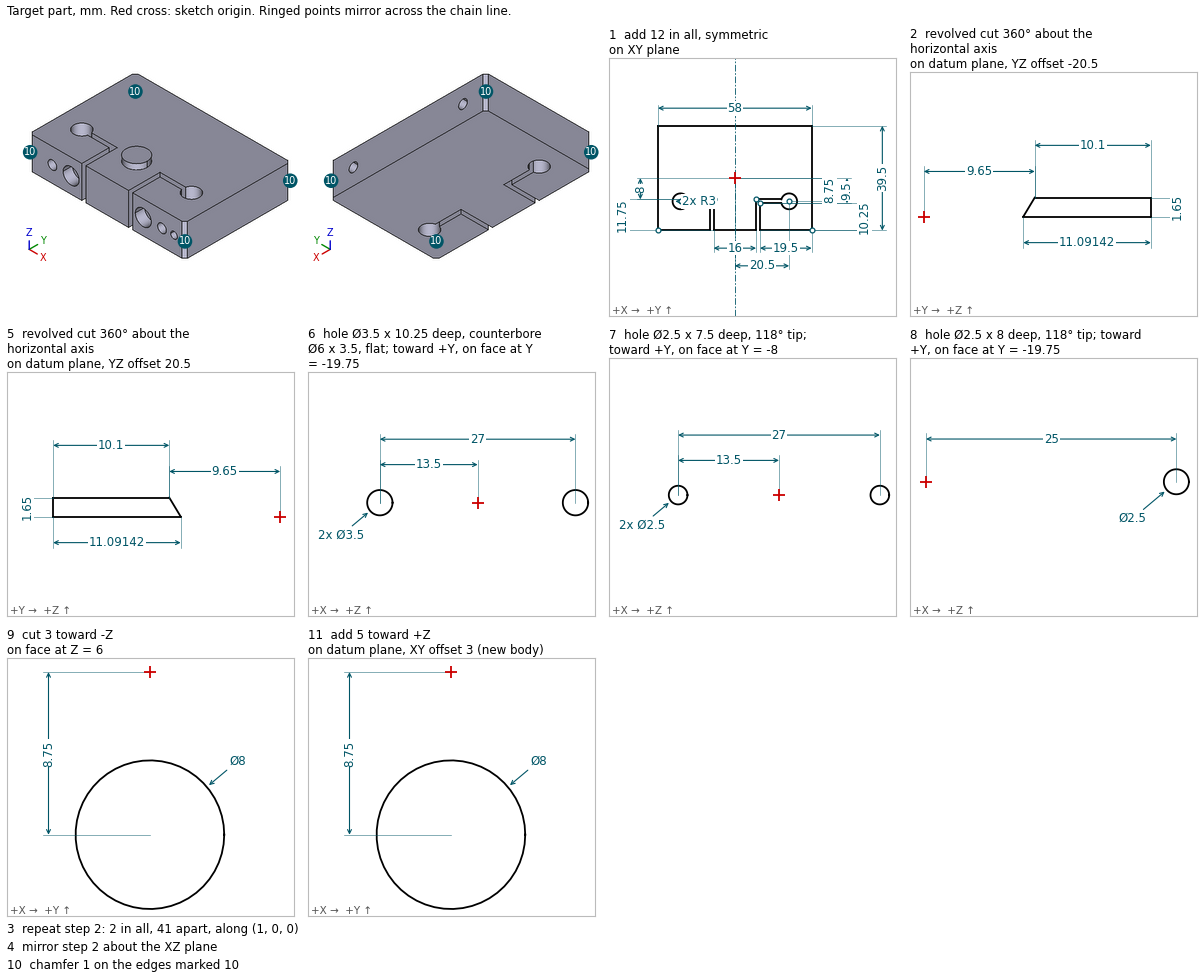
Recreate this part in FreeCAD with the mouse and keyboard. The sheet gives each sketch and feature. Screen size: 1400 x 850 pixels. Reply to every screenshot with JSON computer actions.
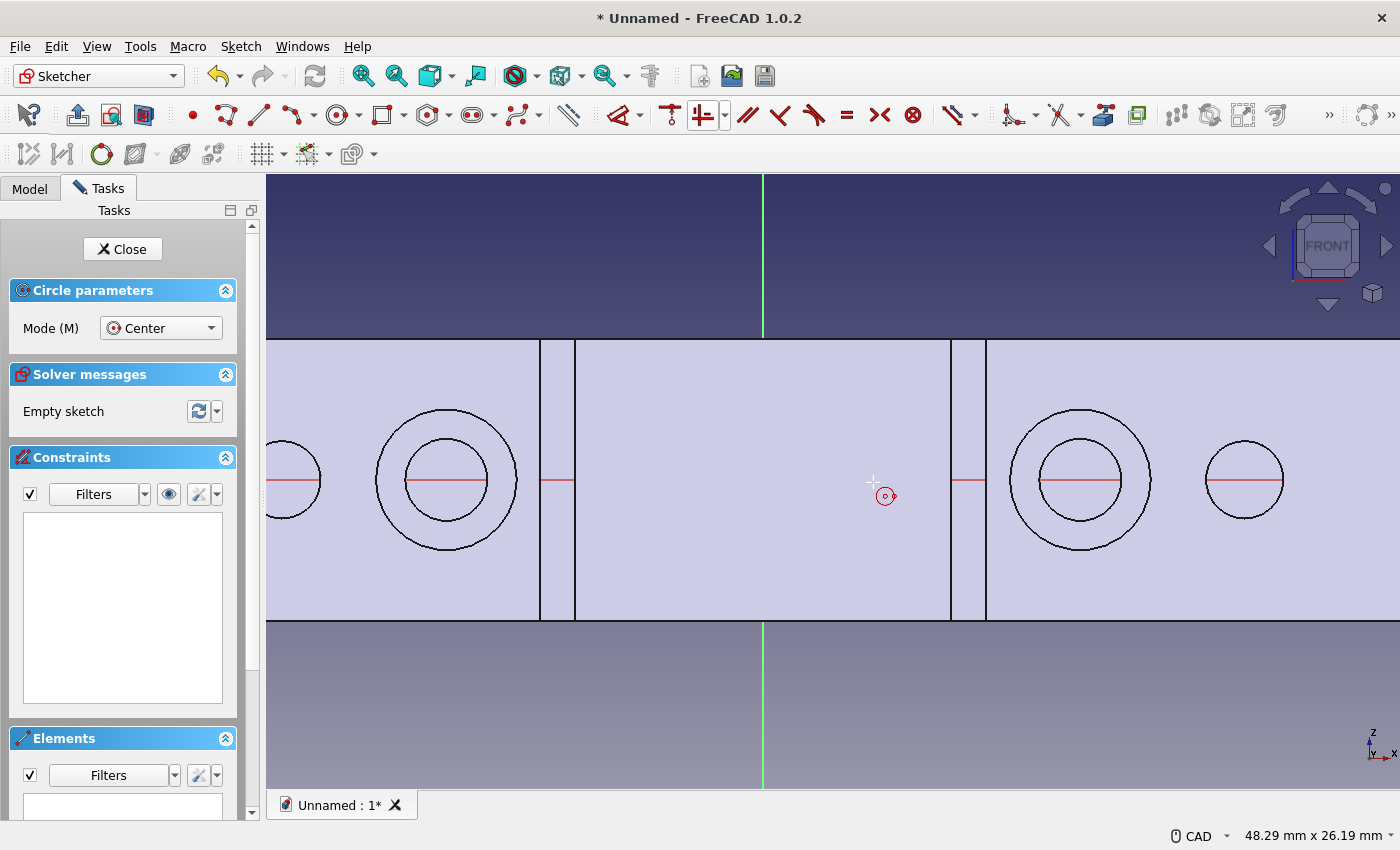
{"action": "left_click", "coordinate": [446, 480]}
{"action": "left_click", "coordinate": [467, 459]}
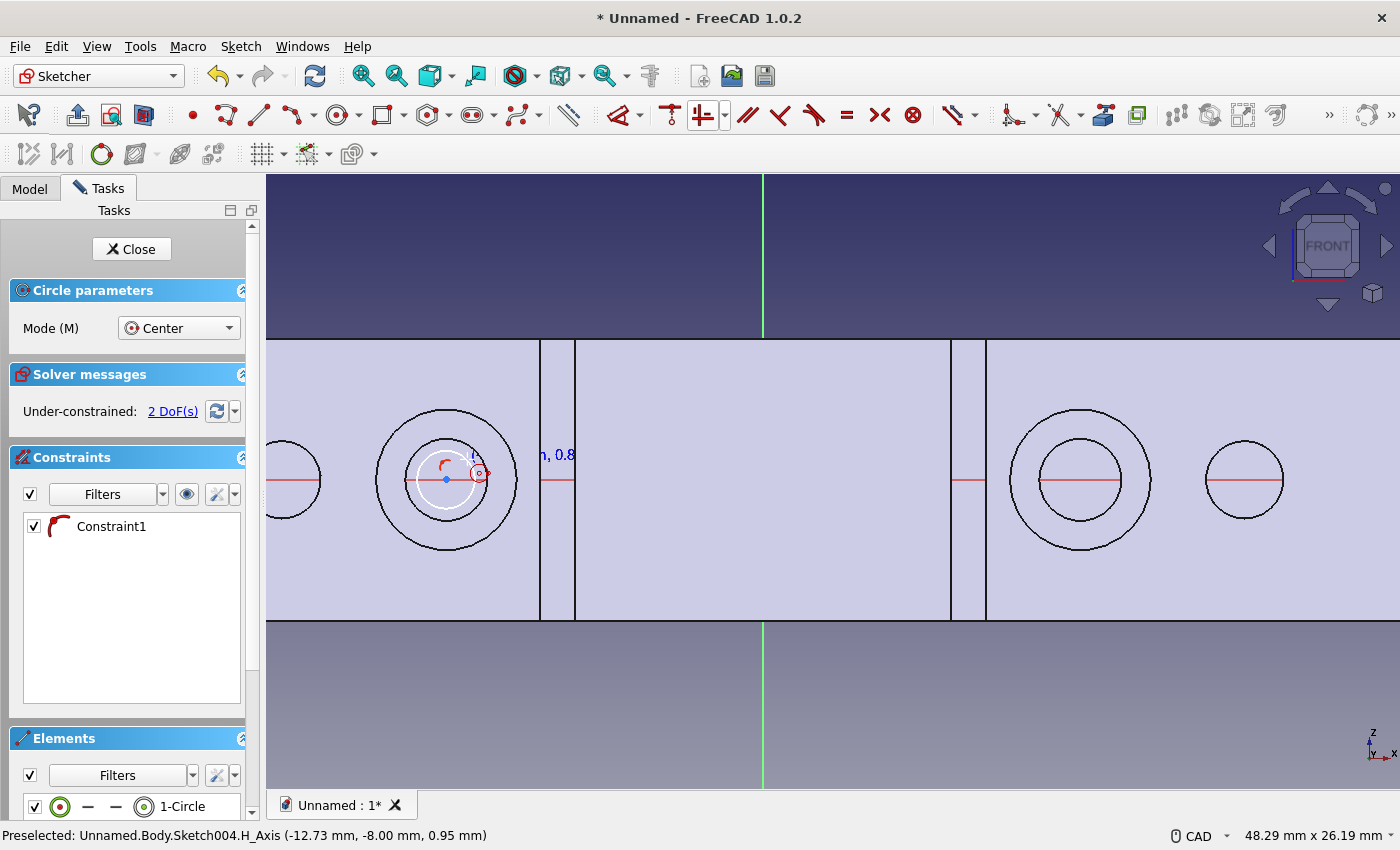
{"action": "left_click", "coordinate": [1080, 480]}
{"action": "left_click", "coordinate": [1101, 459]}
{"action": "key", "text": "Escape"}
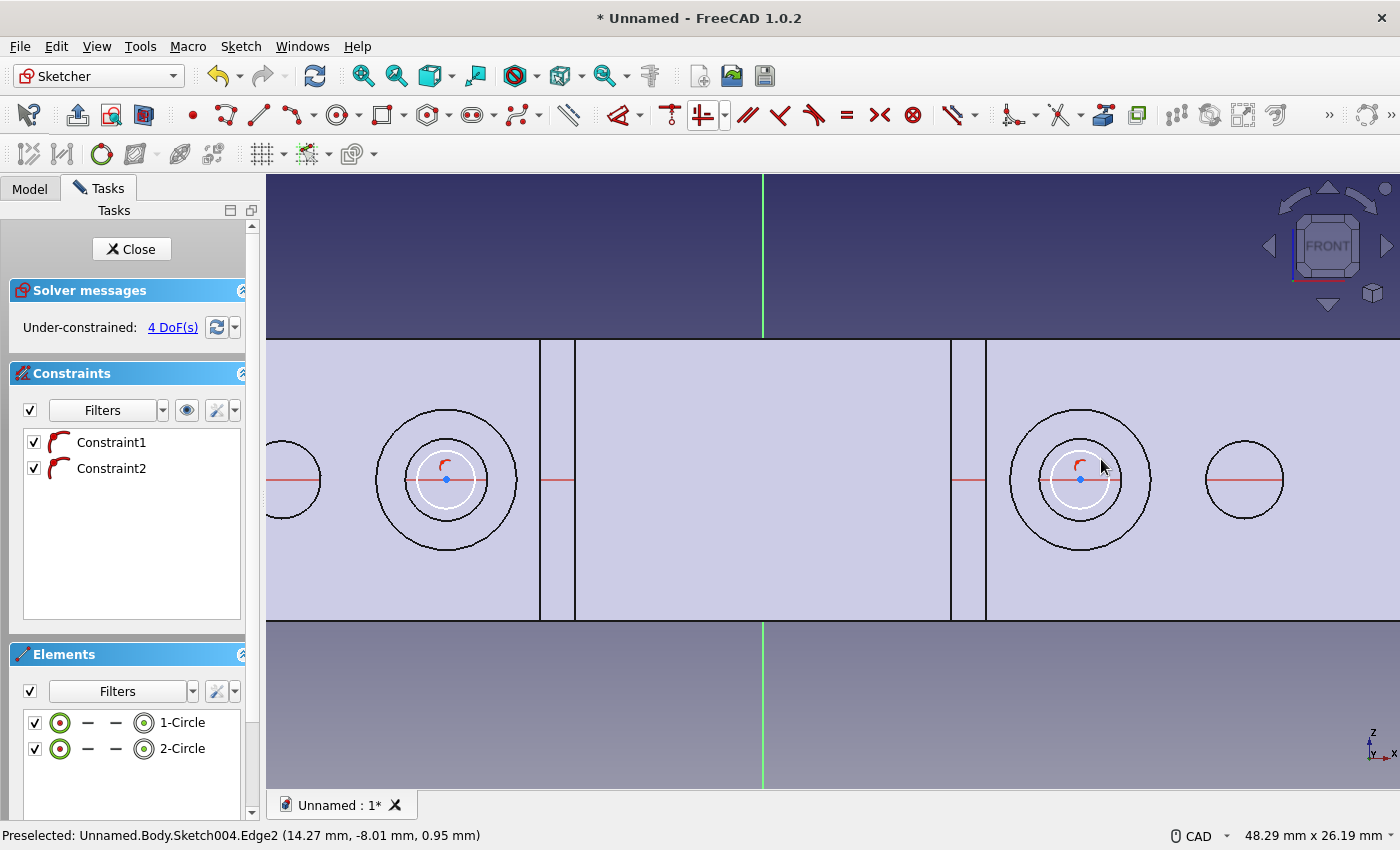
{"action": "left_click", "coordinate": [466, 459]}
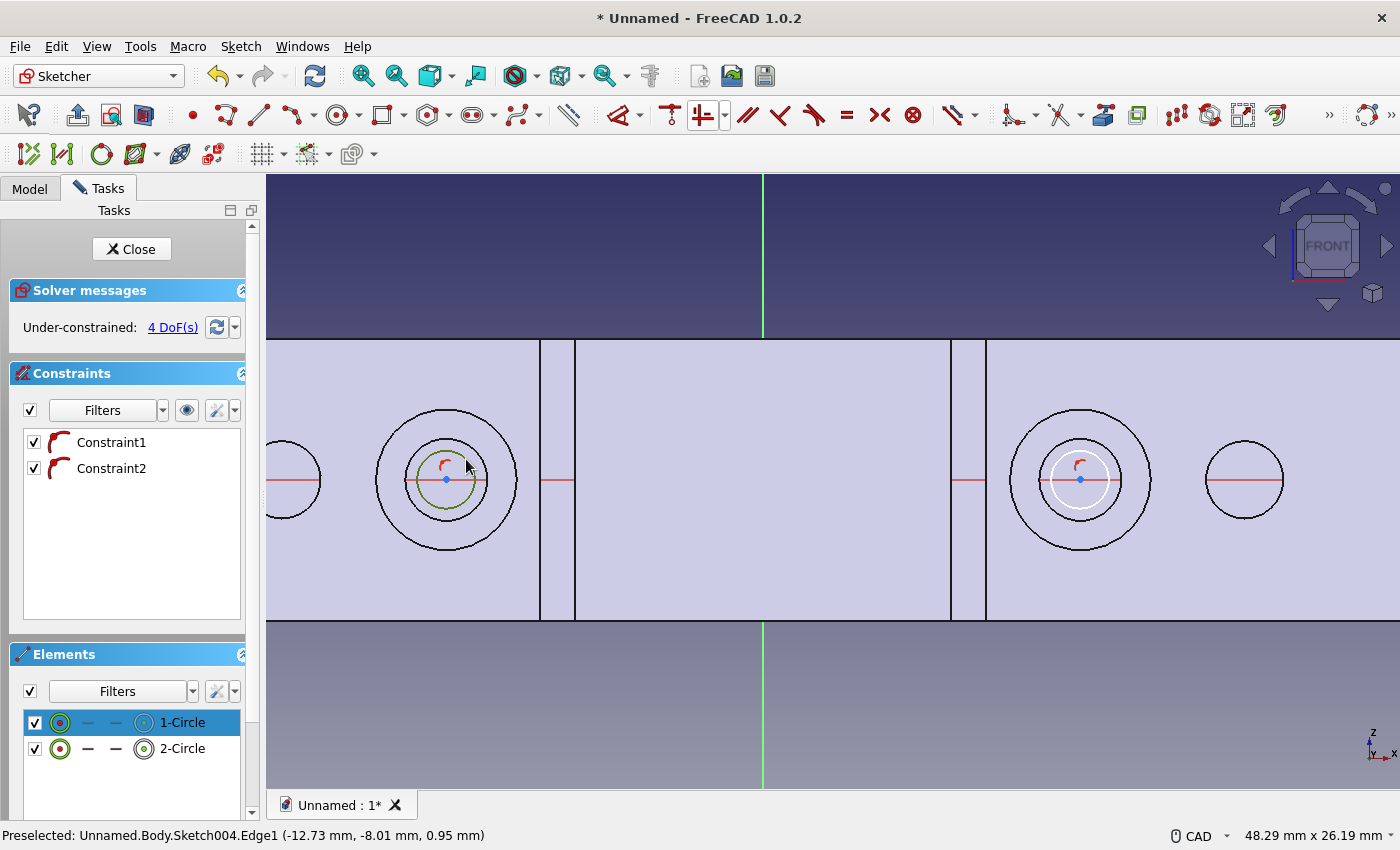
{"action": "left_click", "coordinate": [1100, 459]}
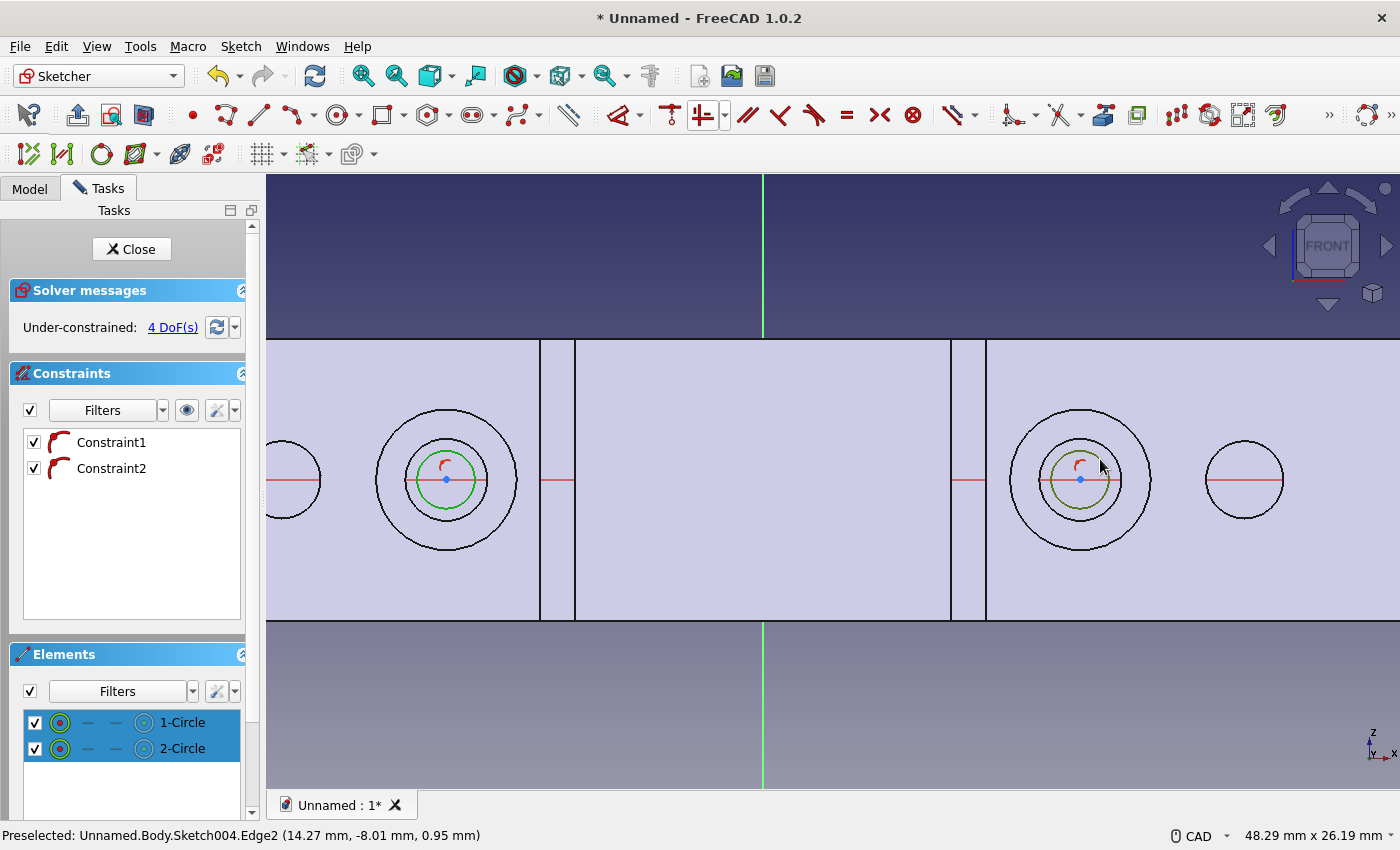
{"action": "left_click", "coordinate": [847, 116]}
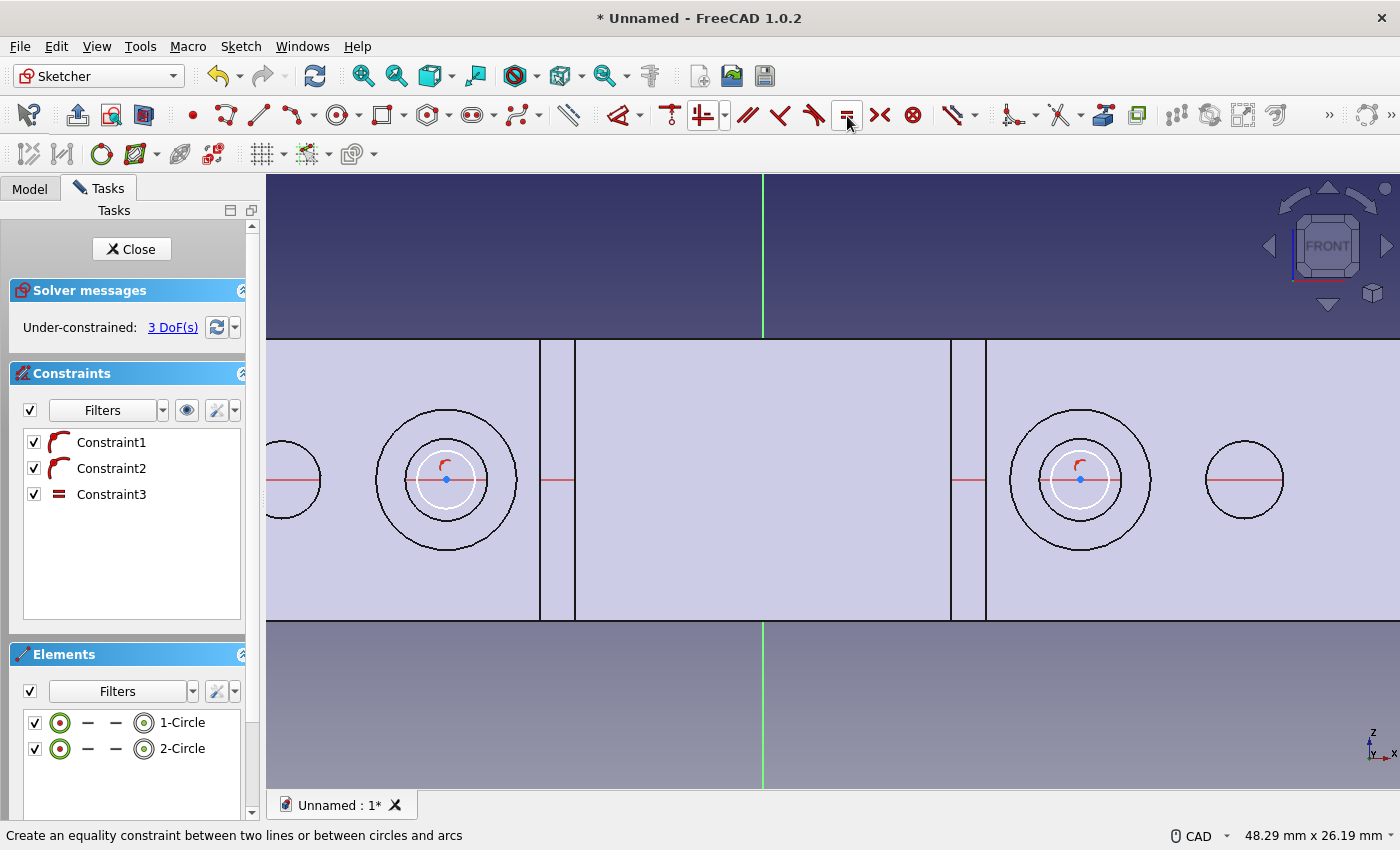
{"action": "left_click", "coordinate": [618, 116]}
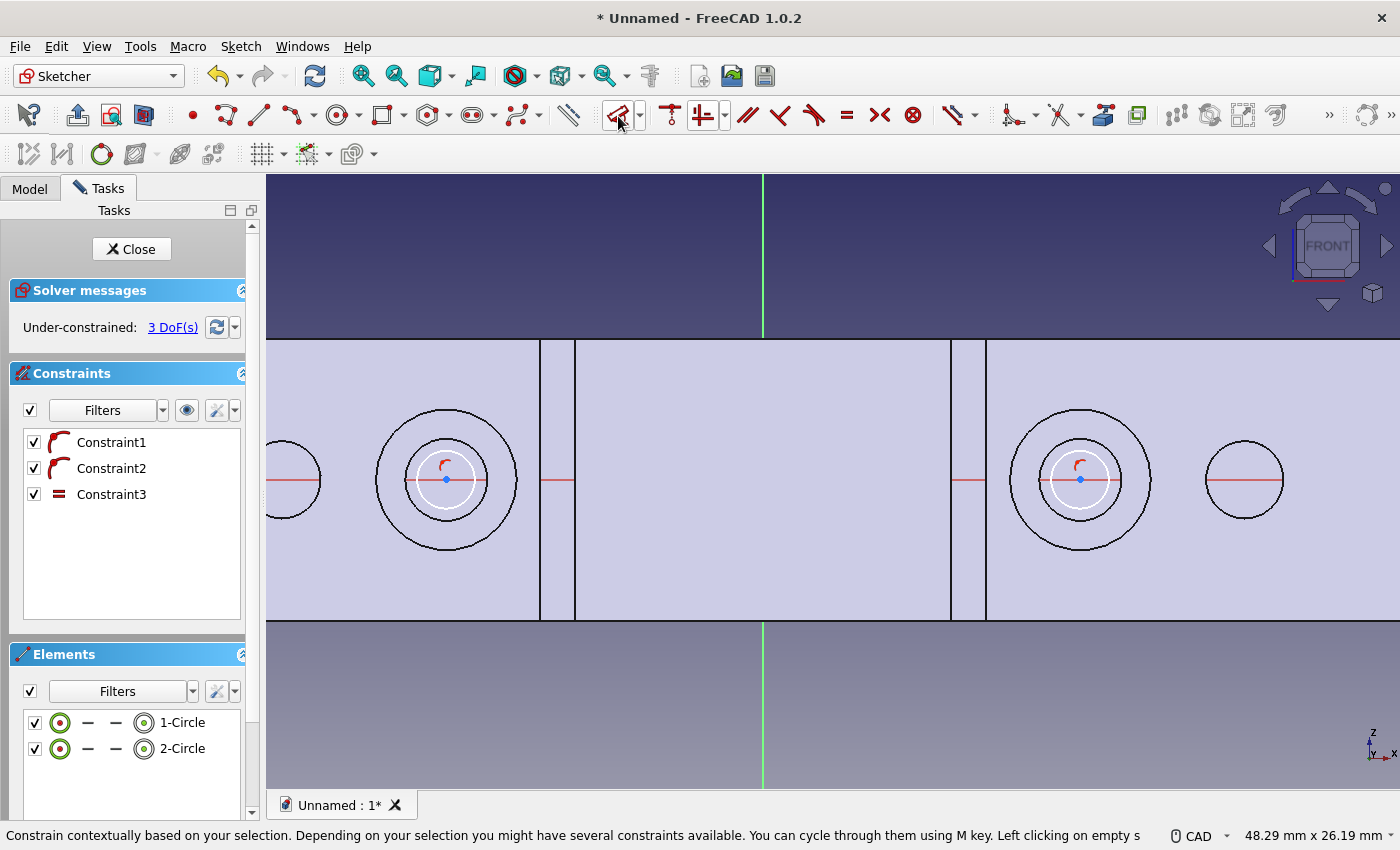
{"action": "left_click", "coordinate": [466, 459]}
{"action": "left_click", "coordinate": [488, 436]}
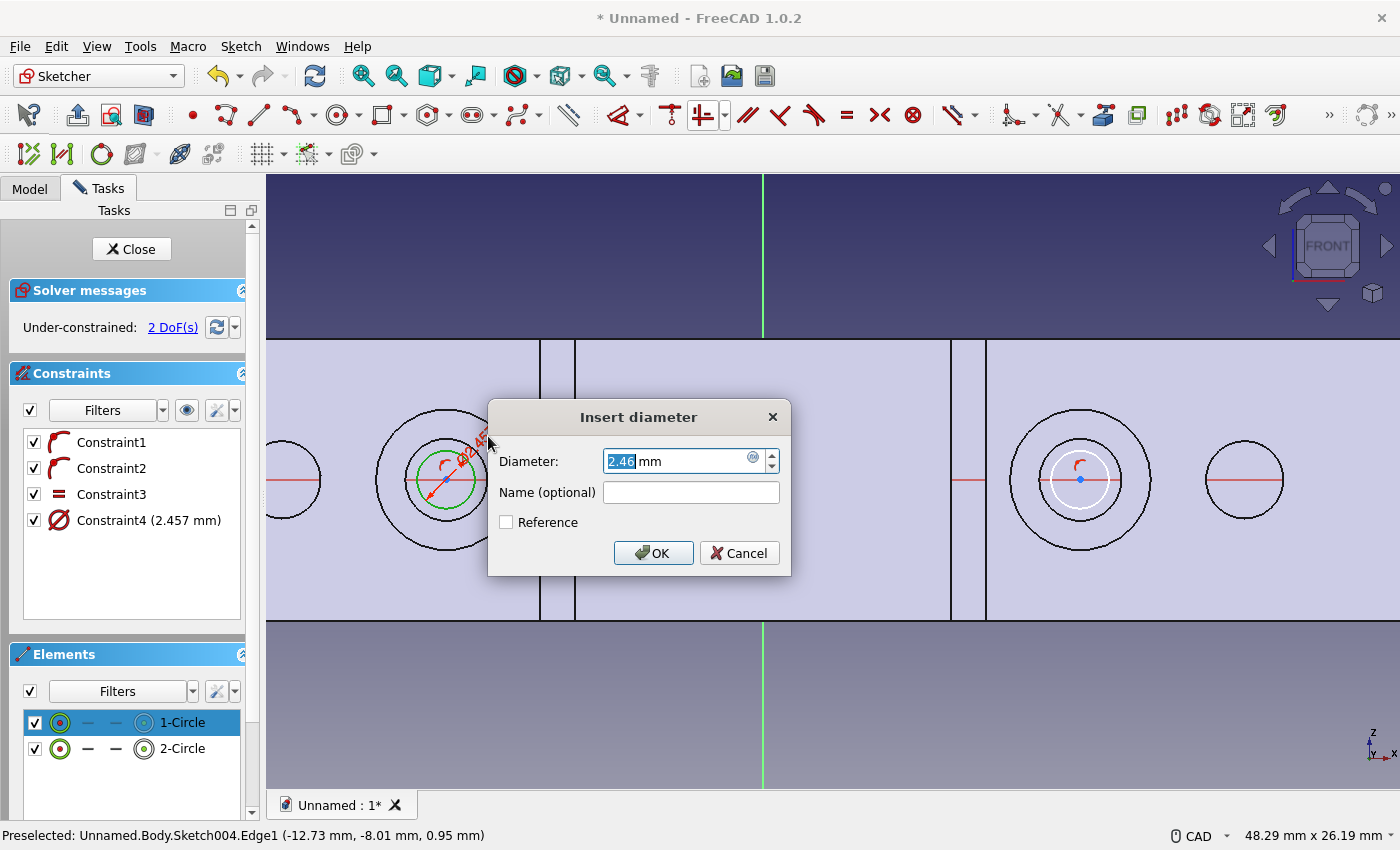
{"action": "type", "text": "2.5"}
{"action": "key", "text": "Return"}